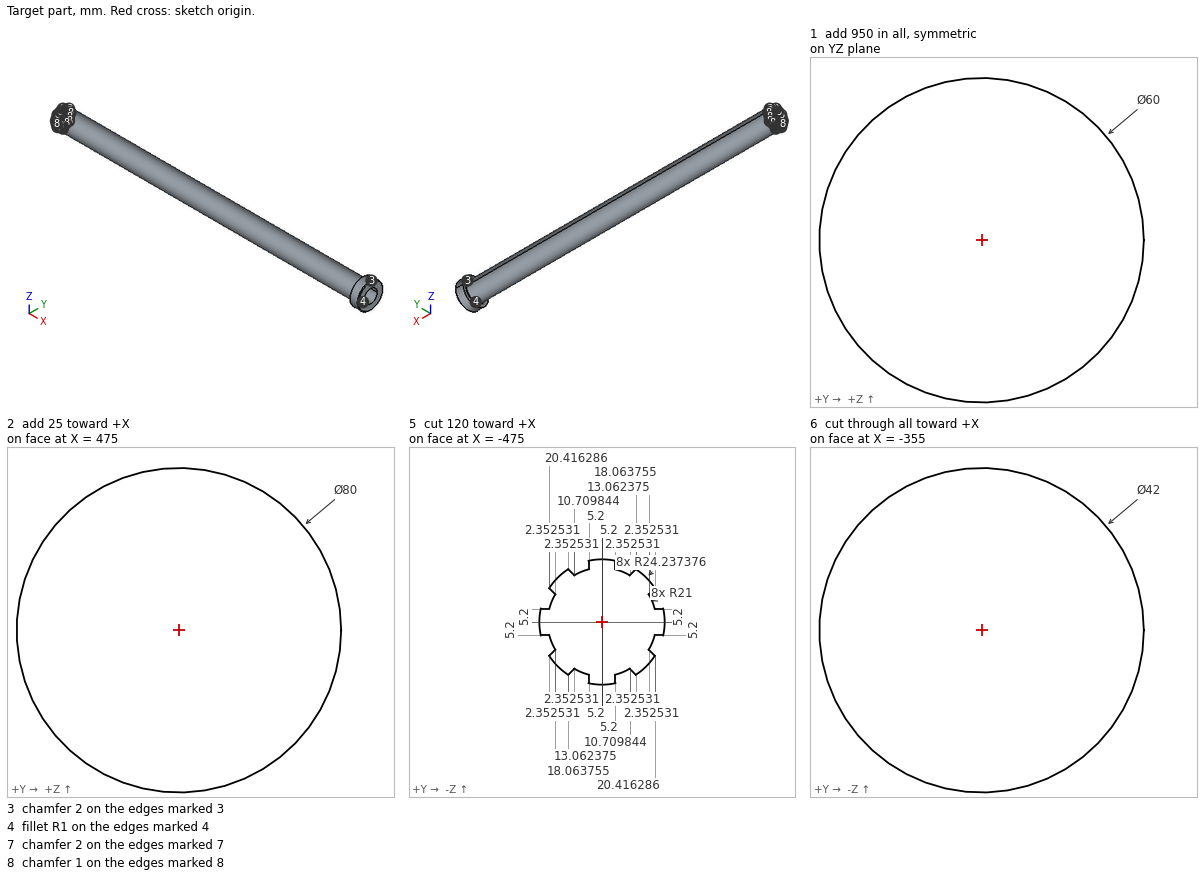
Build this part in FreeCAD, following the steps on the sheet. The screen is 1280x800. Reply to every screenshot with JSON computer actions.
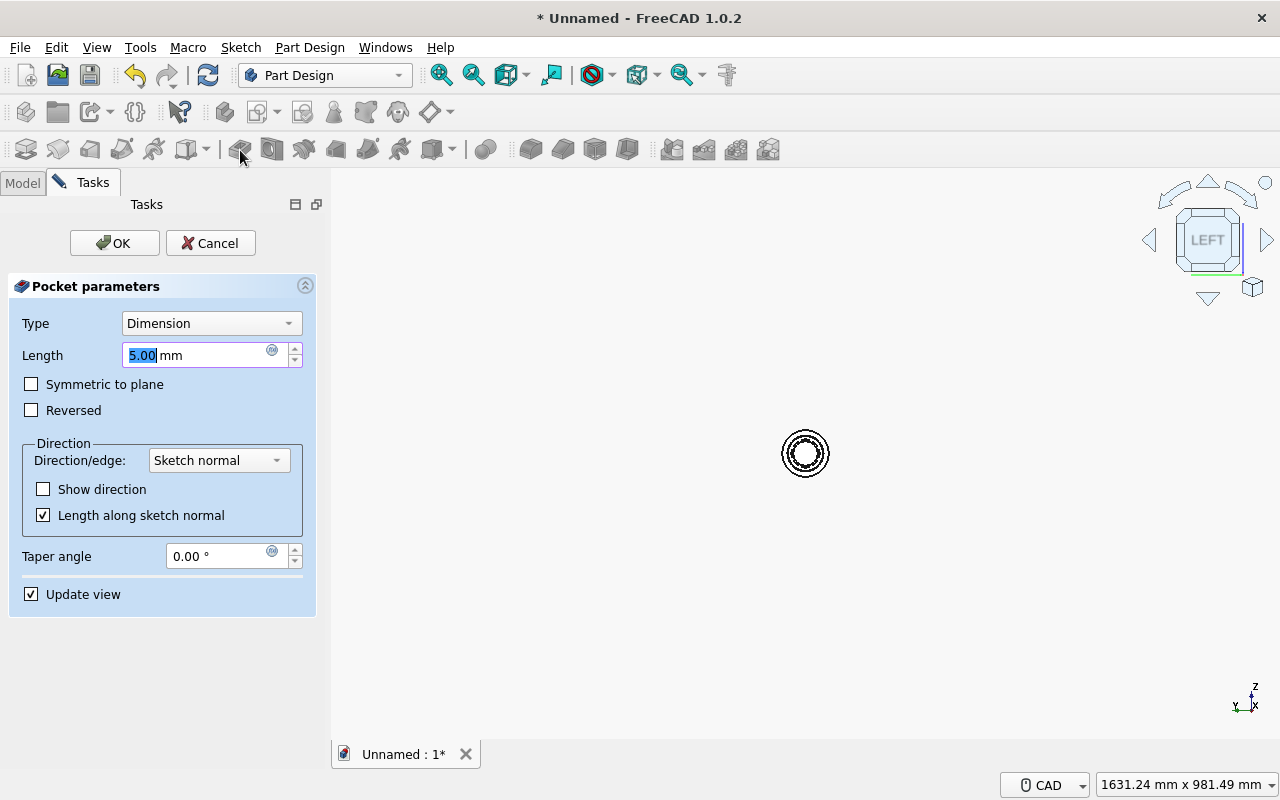
{"action": "left_click", "coordinate": [212, 324]}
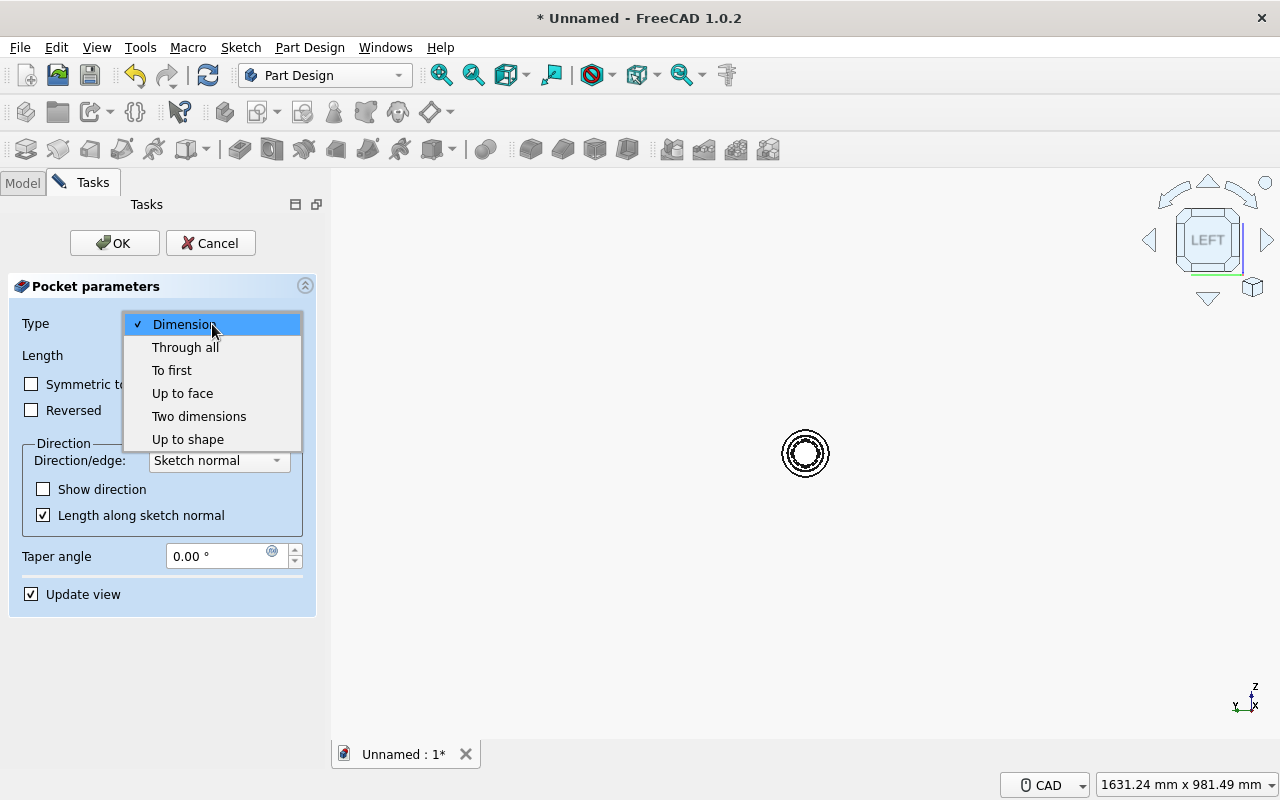
{"action": "left_click", "coordinate": [212, 348]}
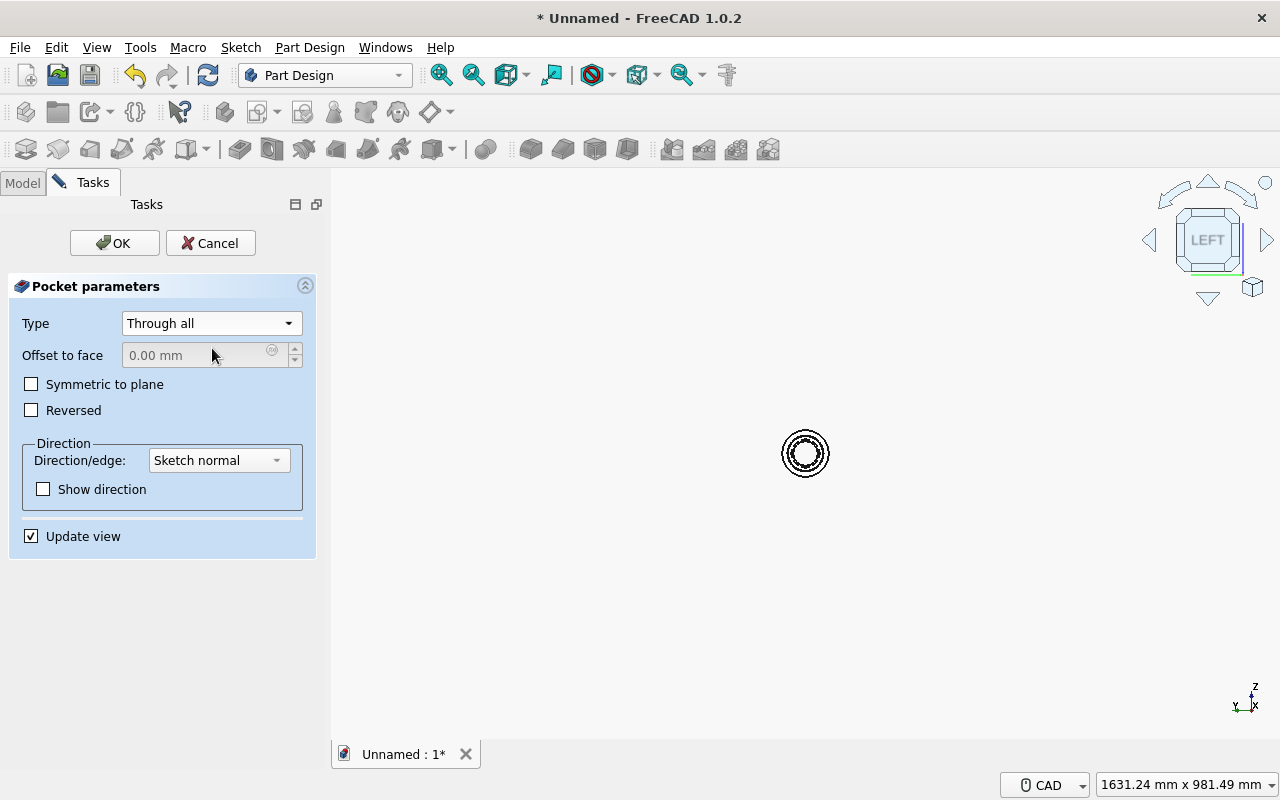
{"action": "left_click", "coordinate": [115, 243]}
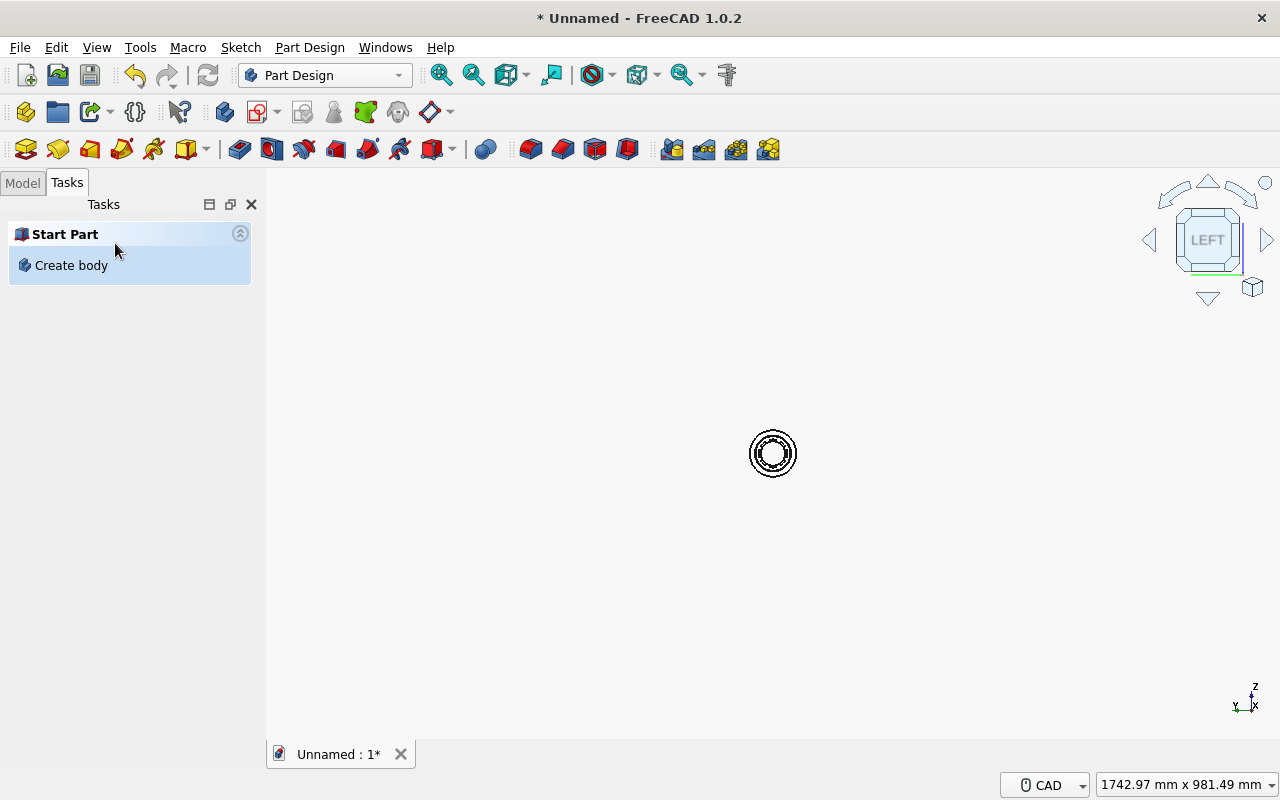
{"action": "key", "text": "v f"}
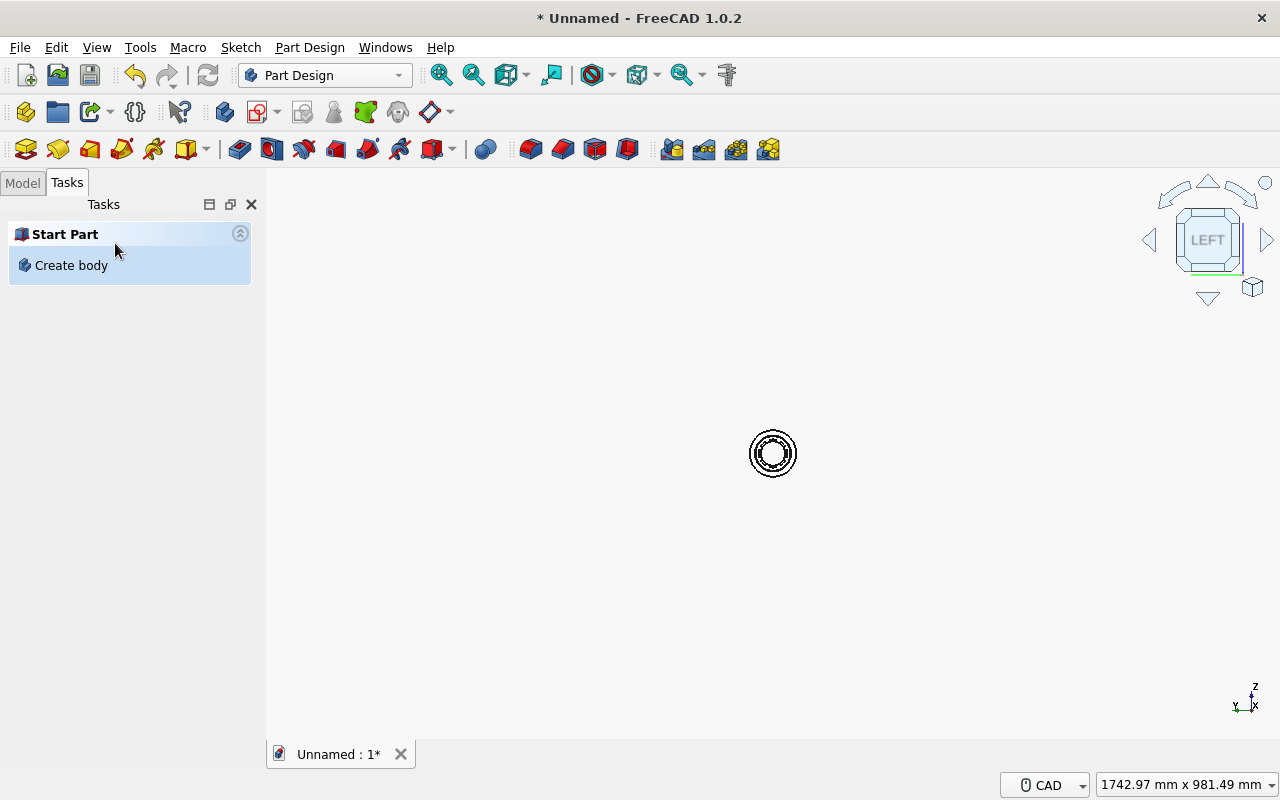
{"action": "key", "text": "0"}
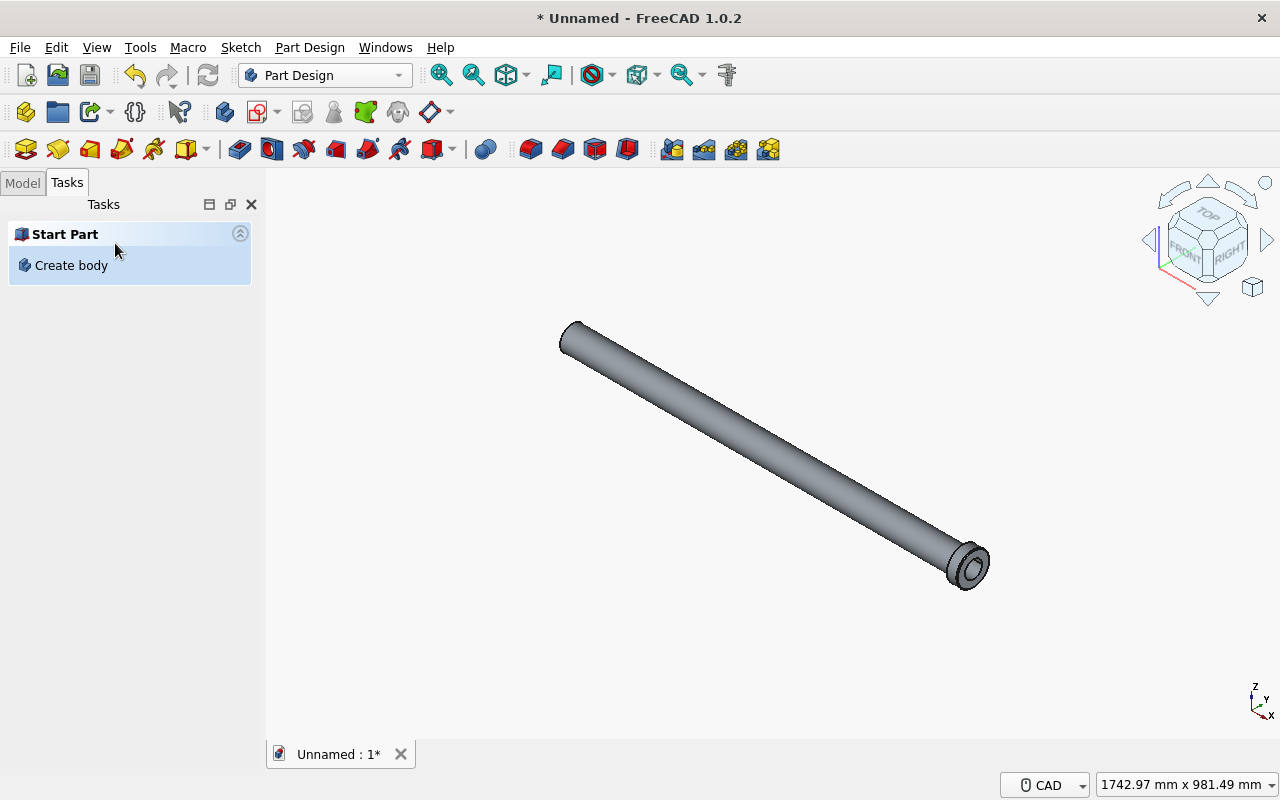
{"action": "left_click", "coordinate": [576, 321]}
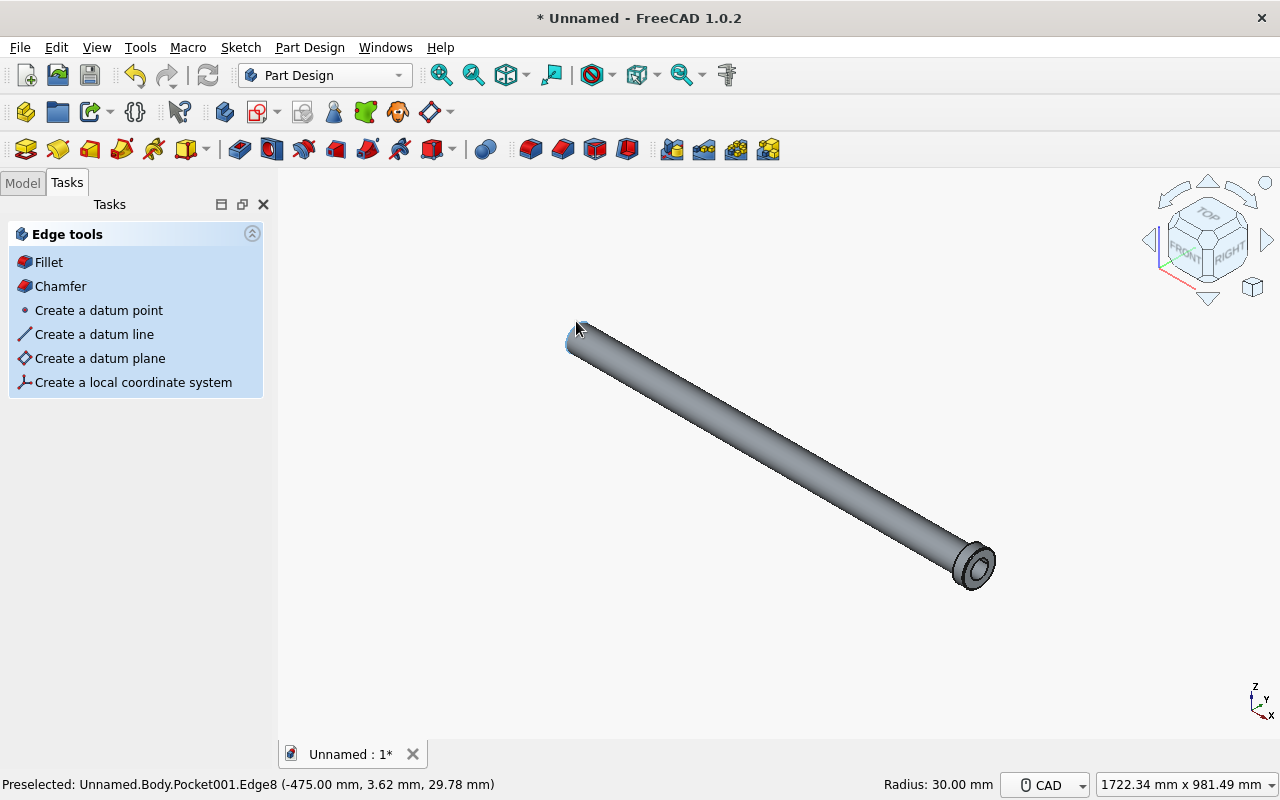
{"action": "left_click", "coordinate": [564, 150]}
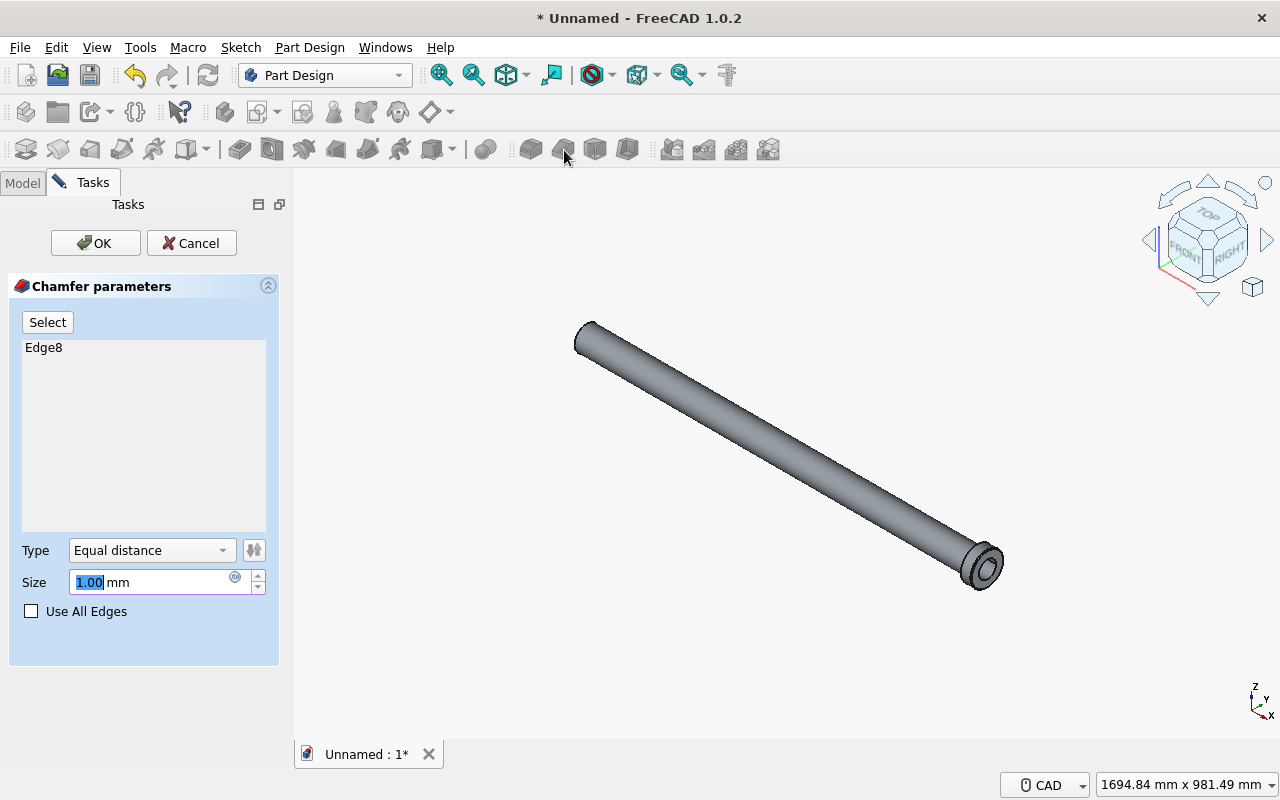
{"action": "type", "text": "2"}
{"action": "key", "text": "Tab"}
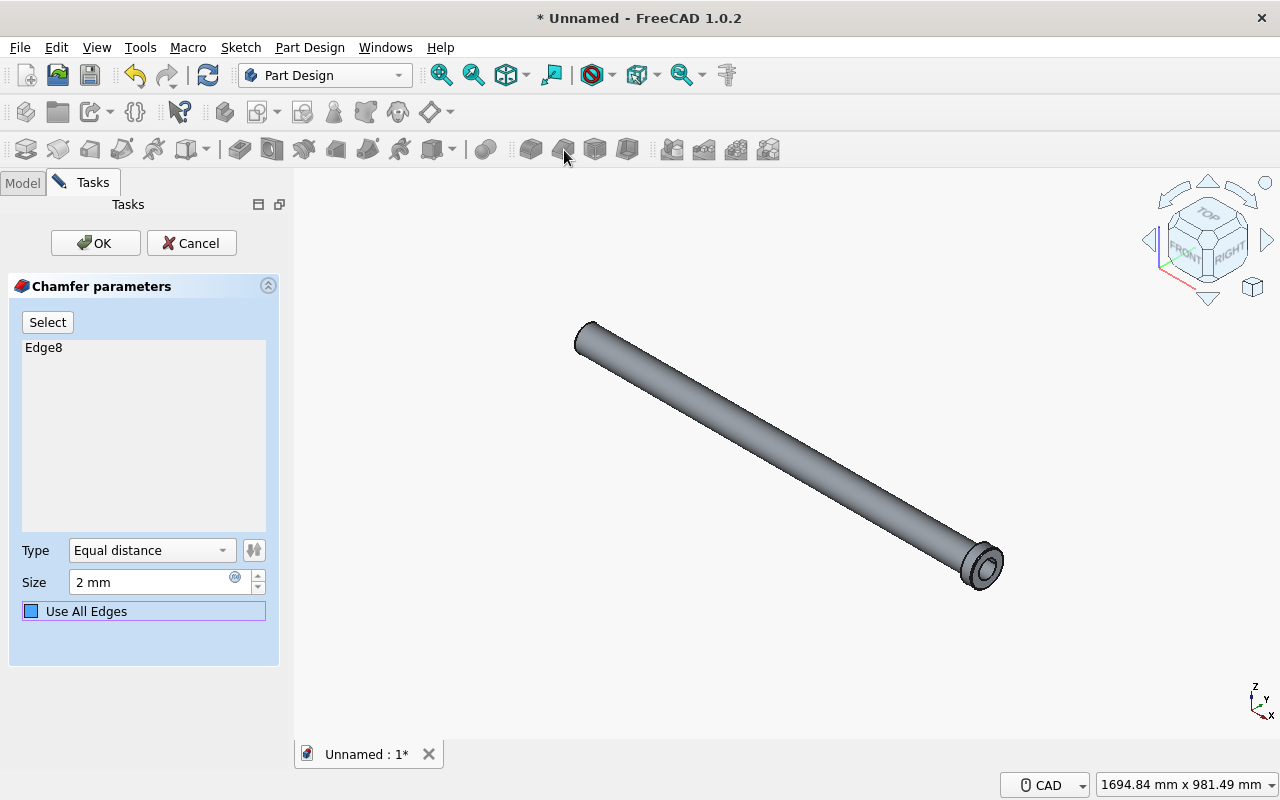
{"action": "left_click", "coordinate": [96, 243]}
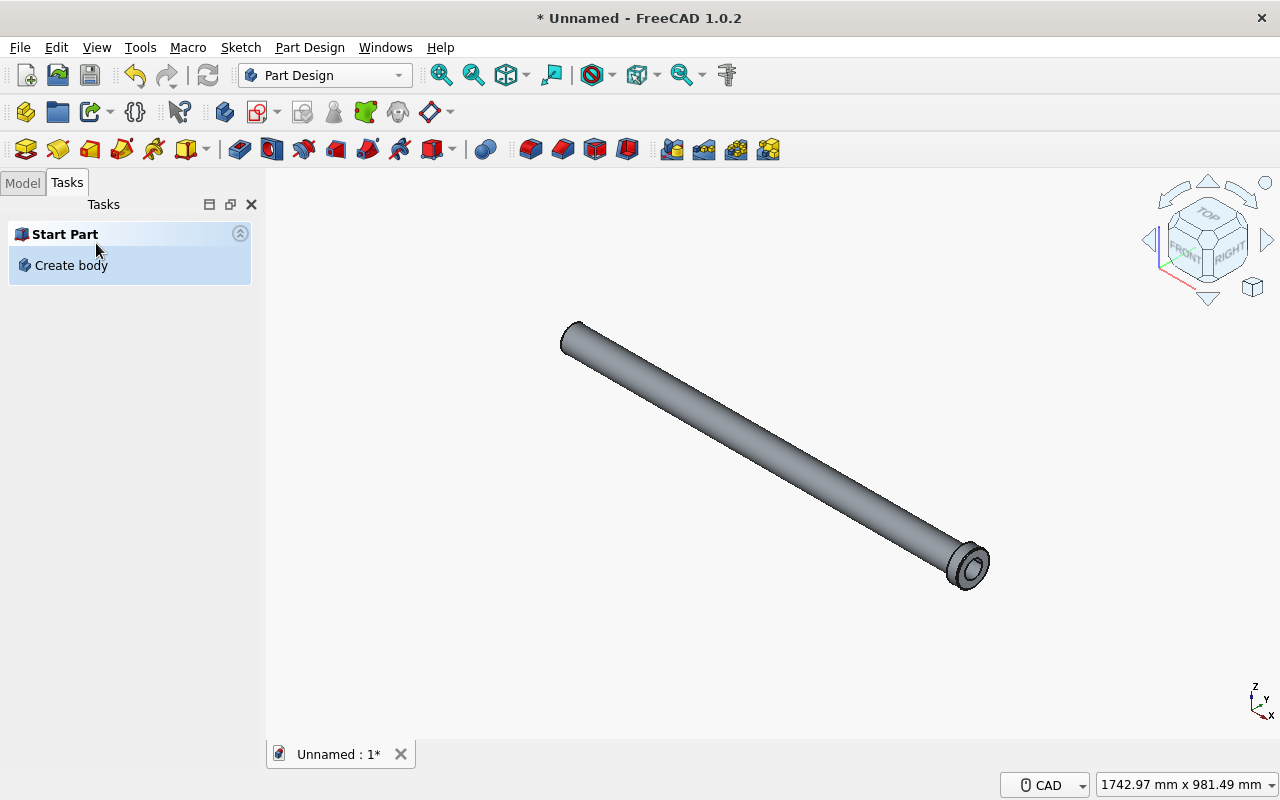
{"action": "scroll", "coordinate": [562, 342], "scroll_direction": "up", "scroll_amount": 10}